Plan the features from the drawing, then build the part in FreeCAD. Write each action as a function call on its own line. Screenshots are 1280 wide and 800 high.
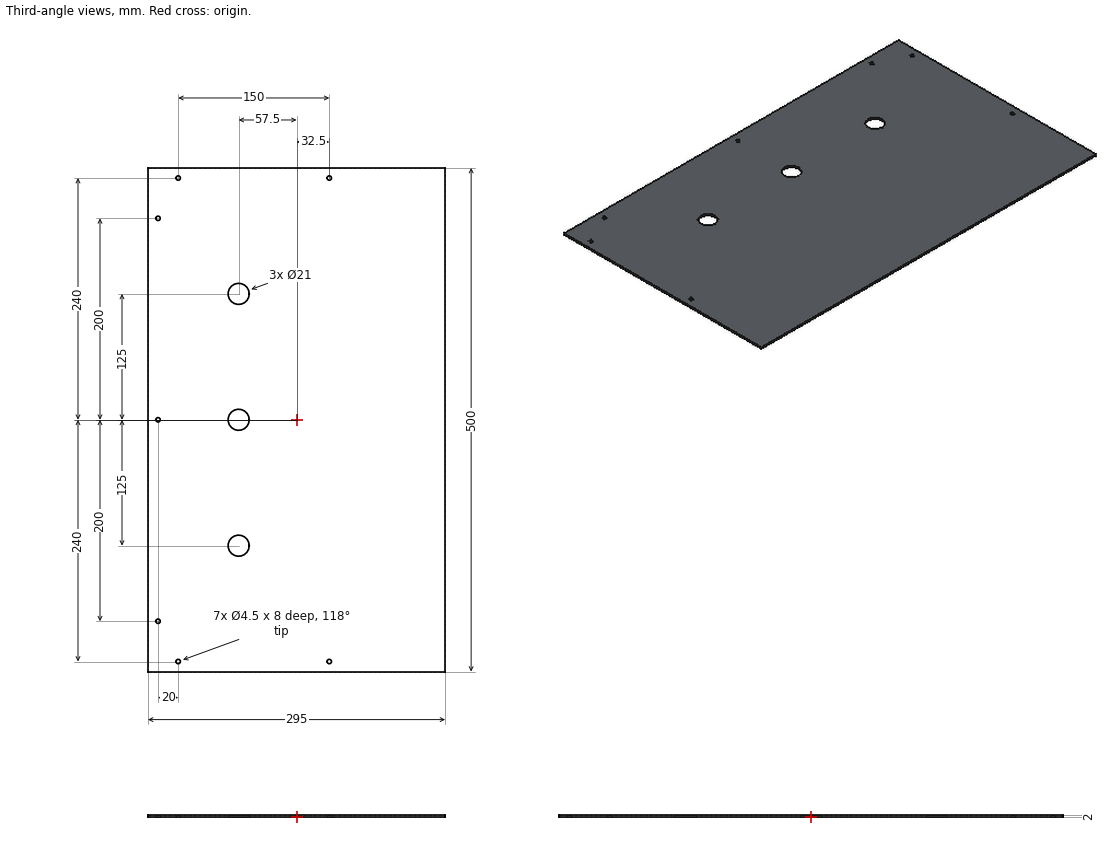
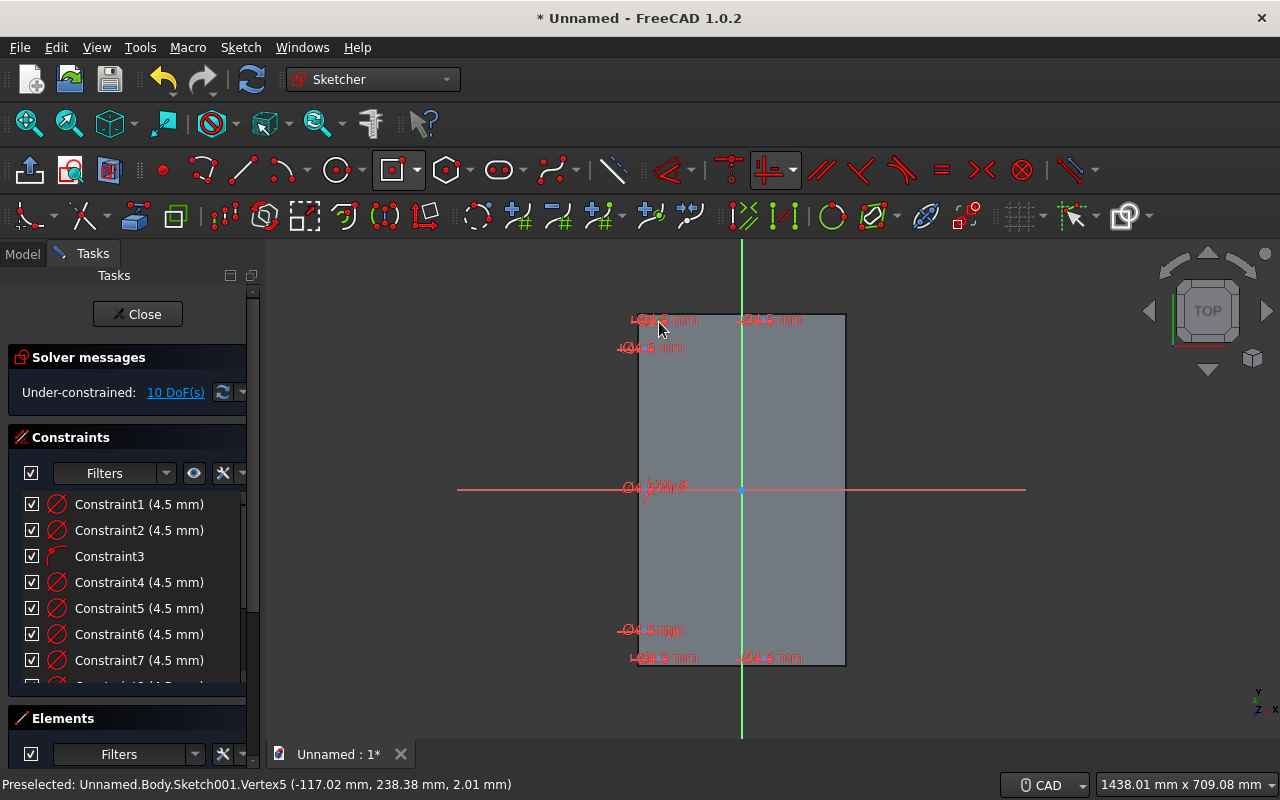
click(764, 322)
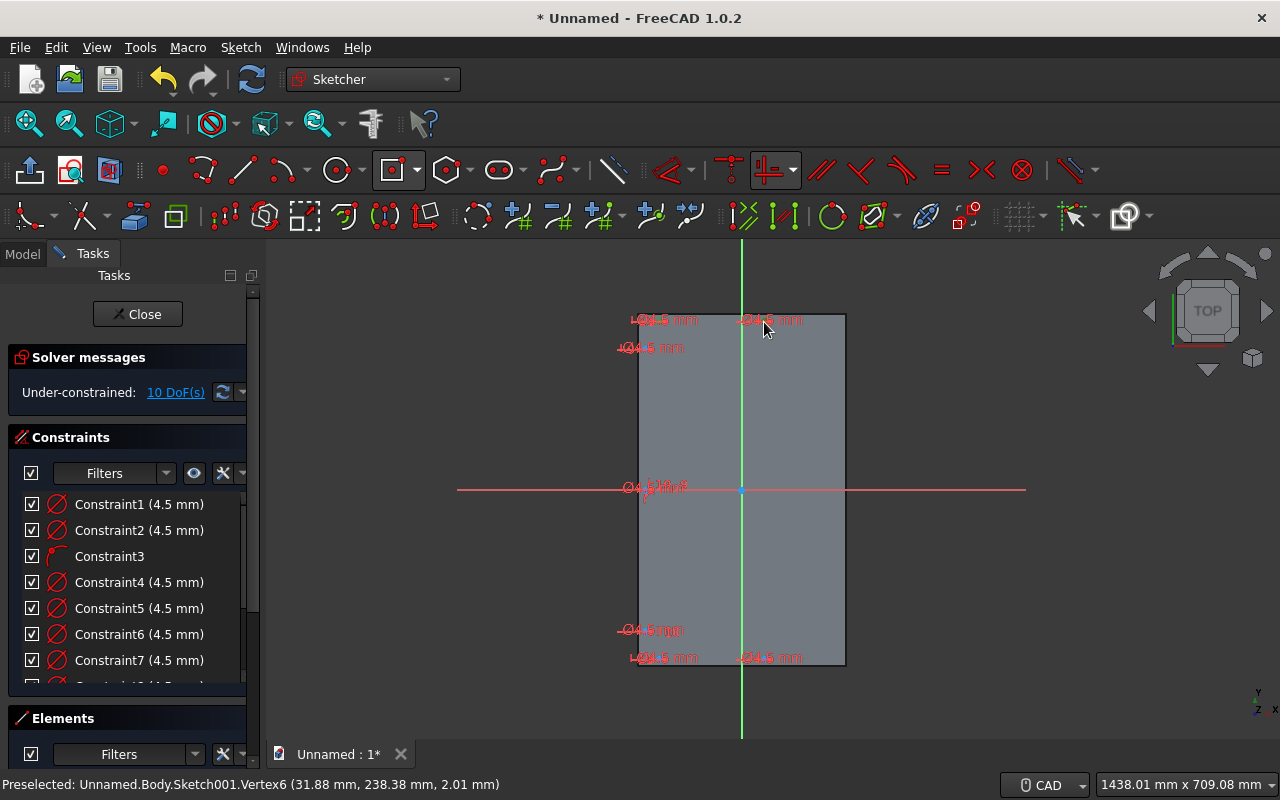
key(h)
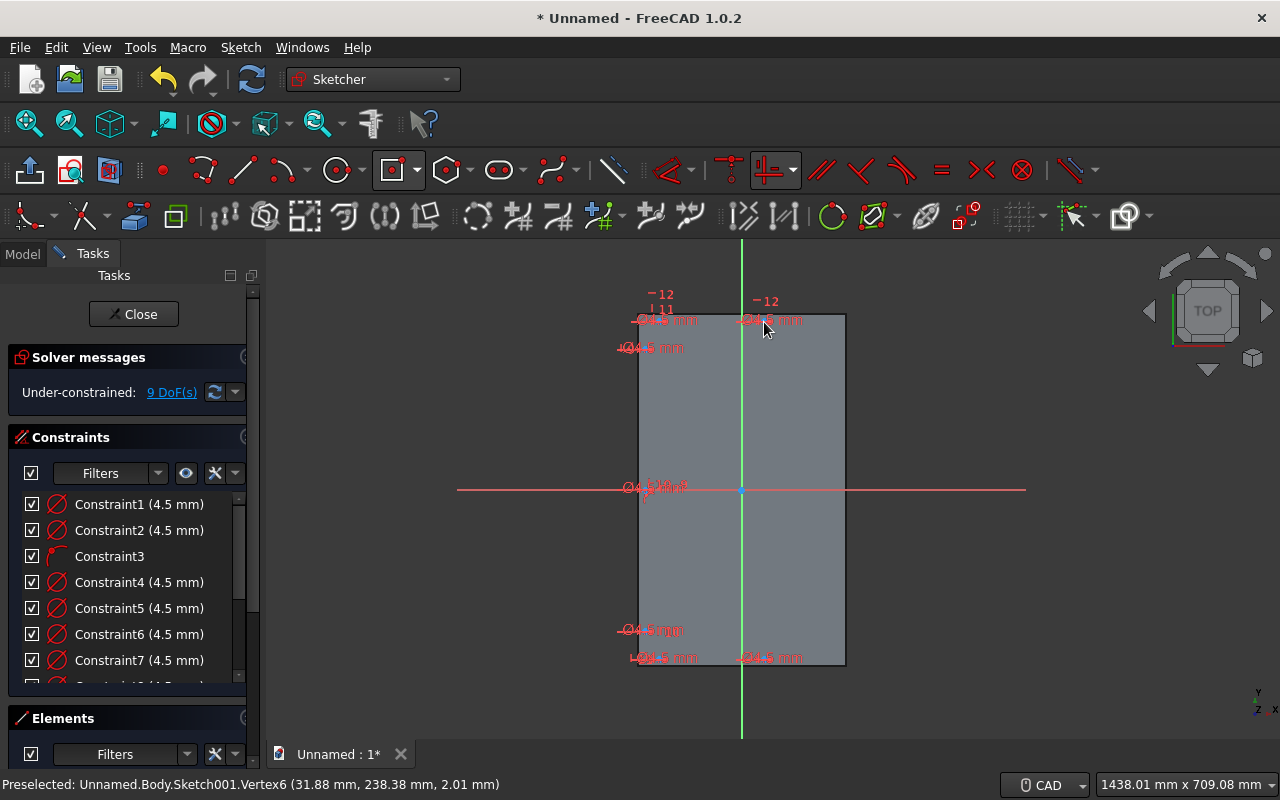
click(764, 322)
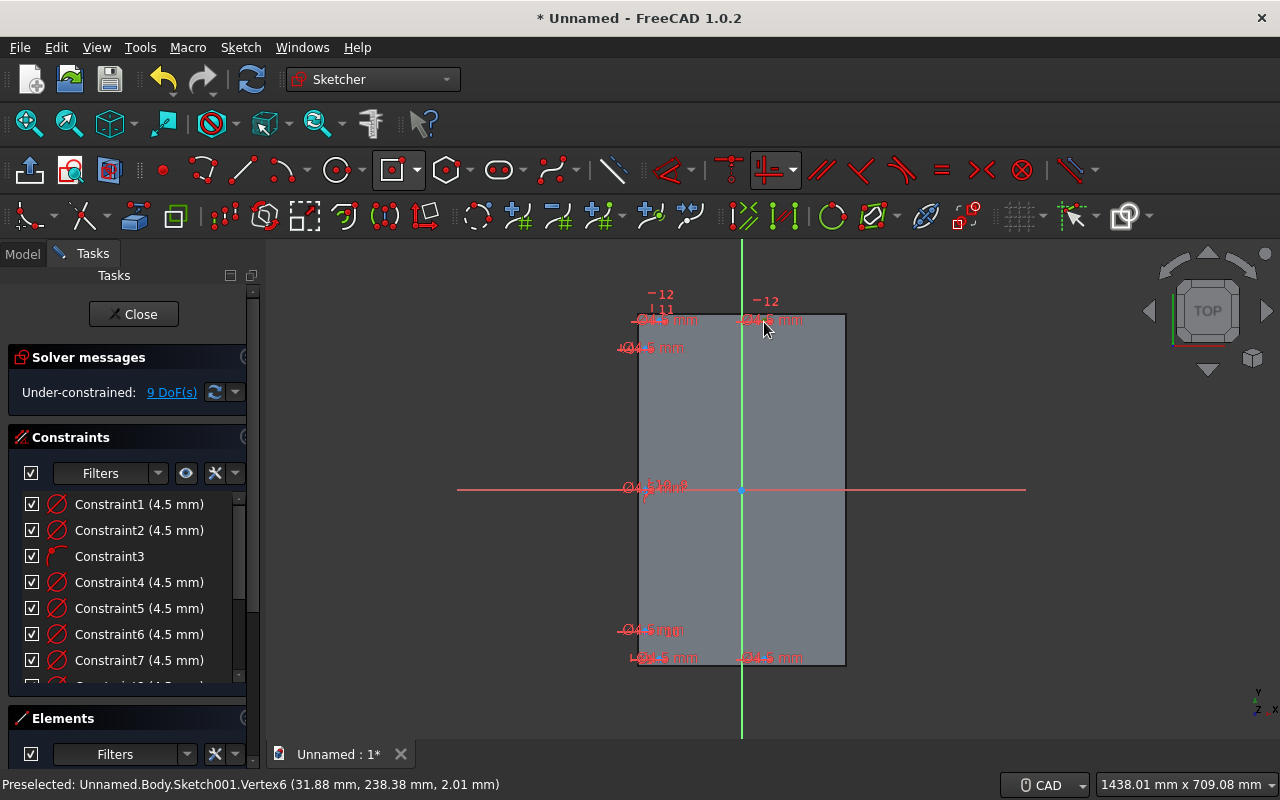
click(764, 660)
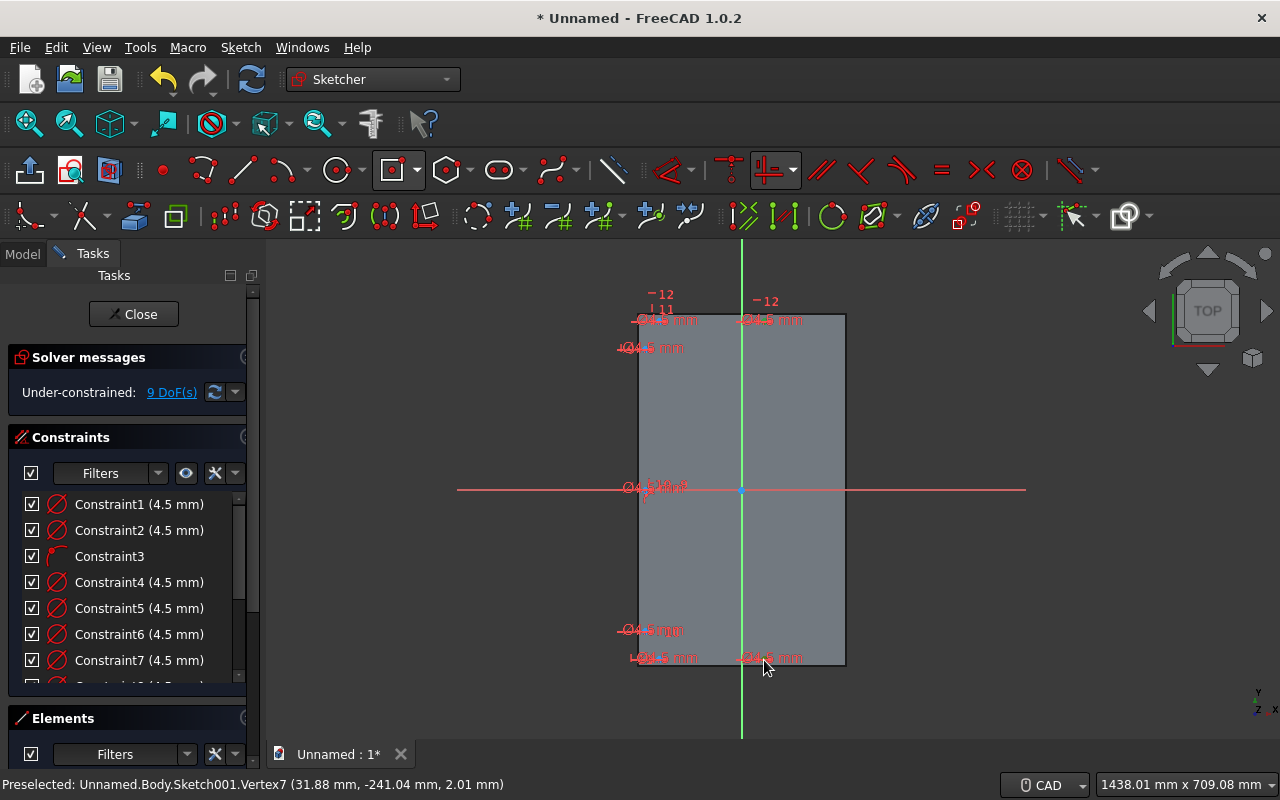
click(796, 170)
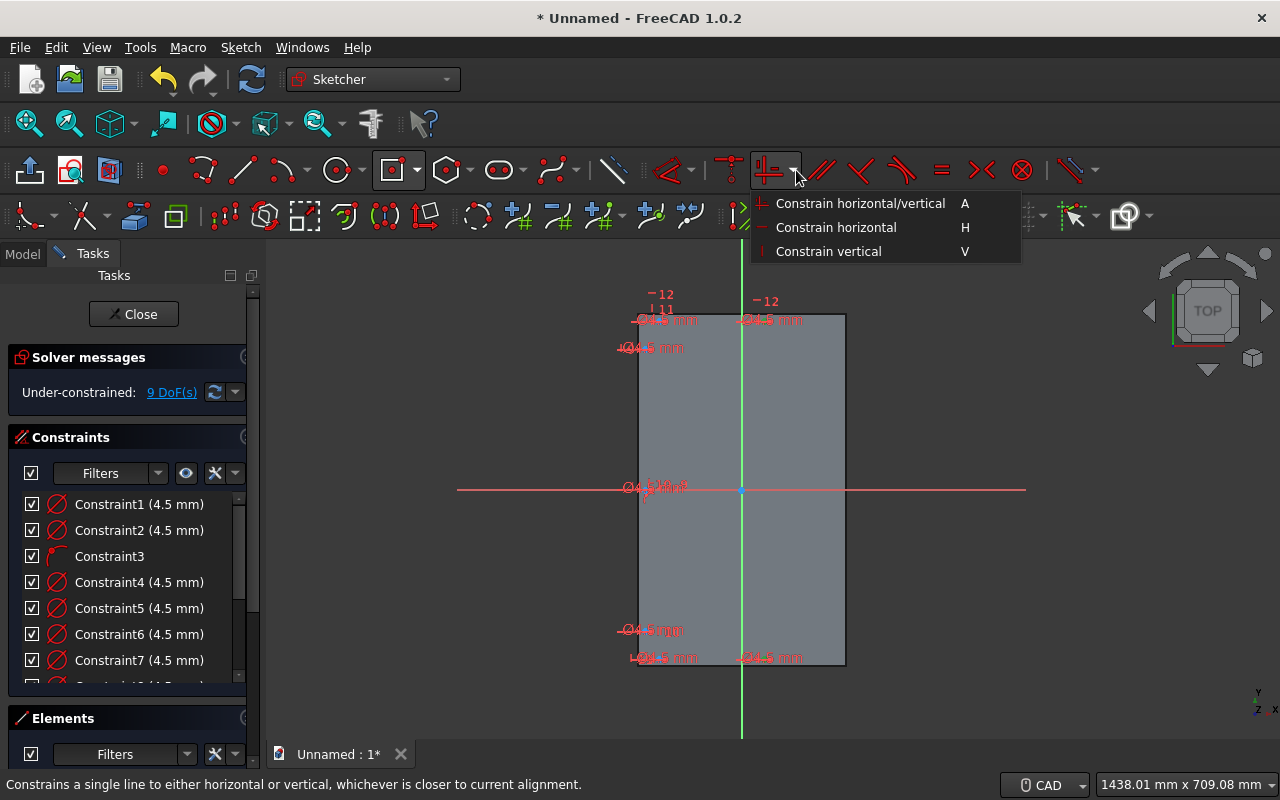
click(886, 251)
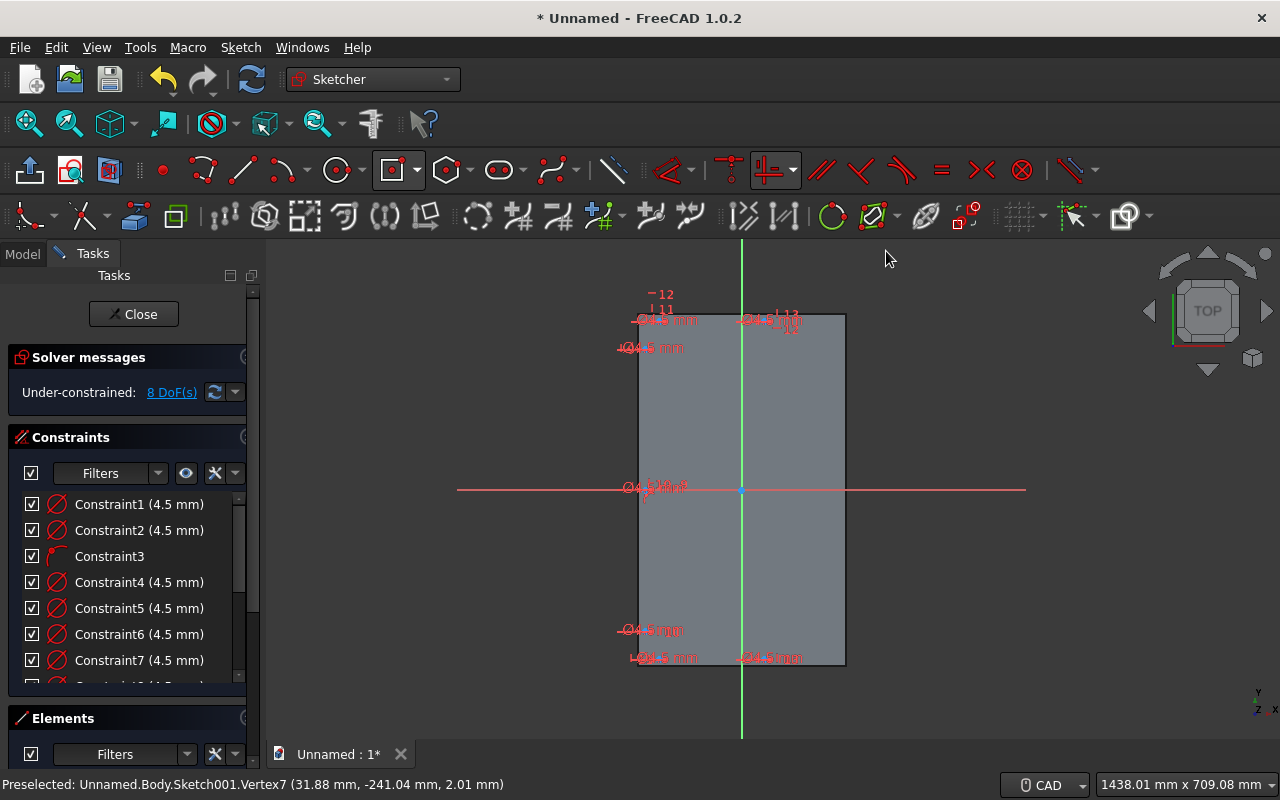
click(659, 660)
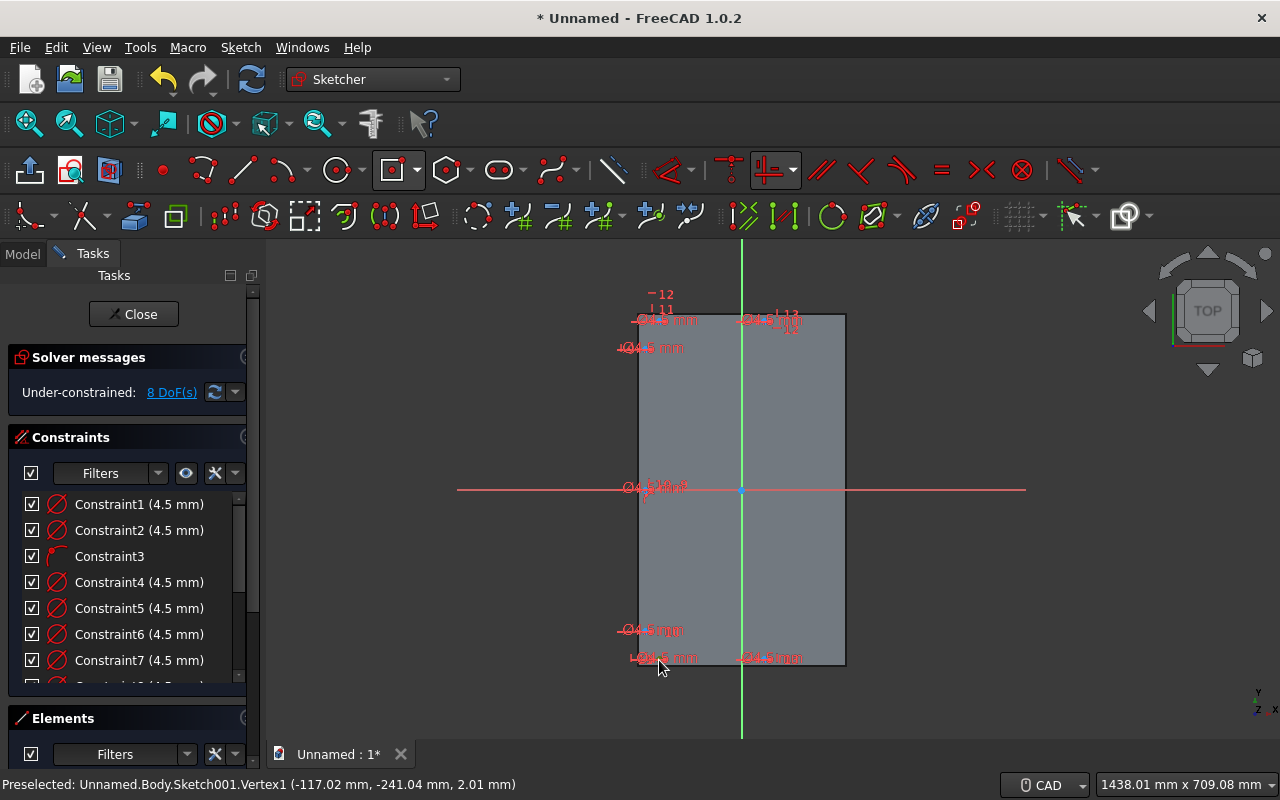
click(764, 660)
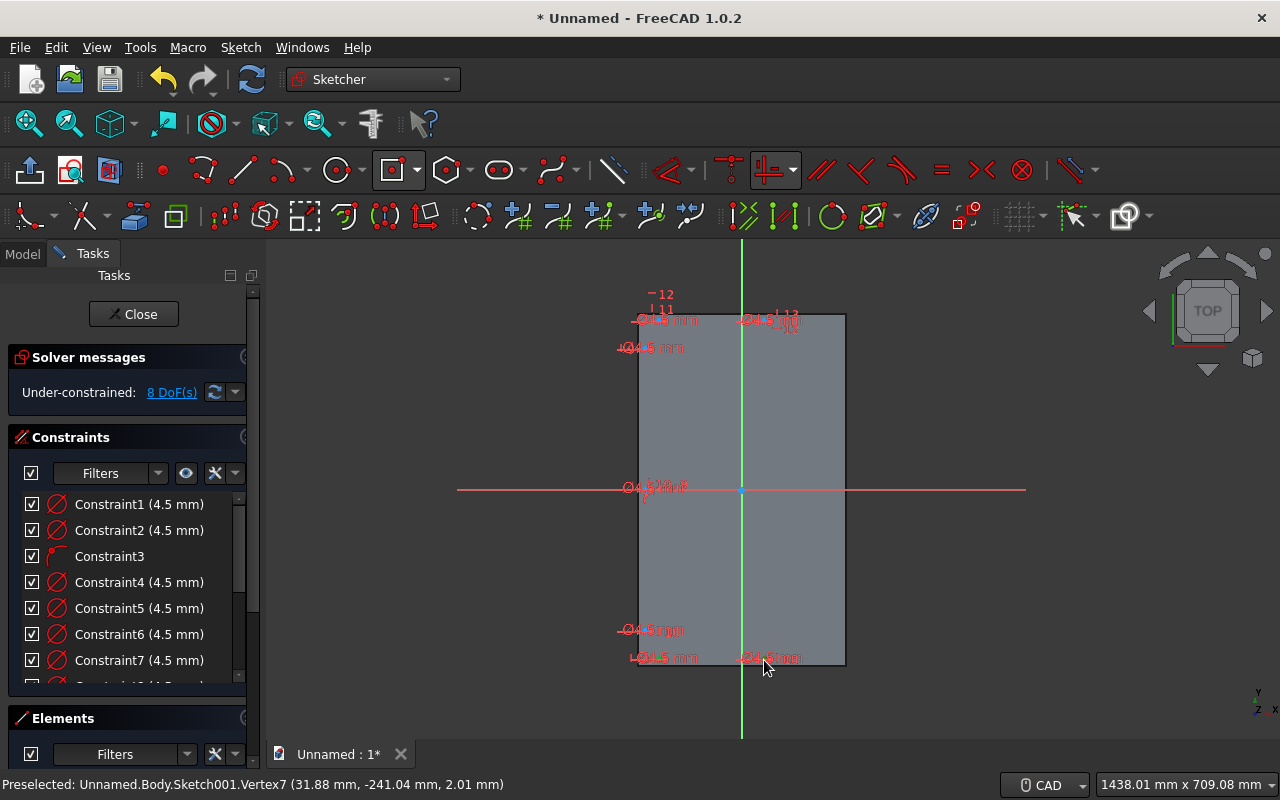
key(h)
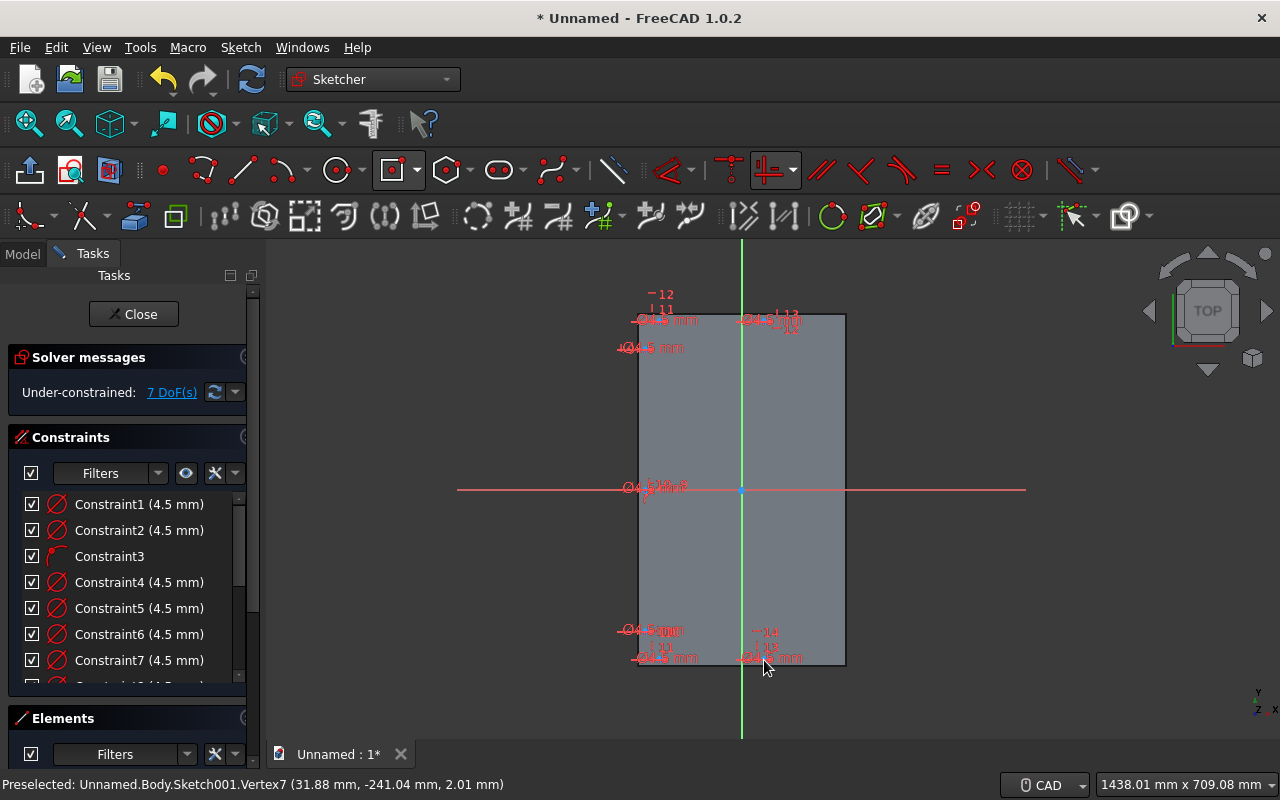
click(659, 660)